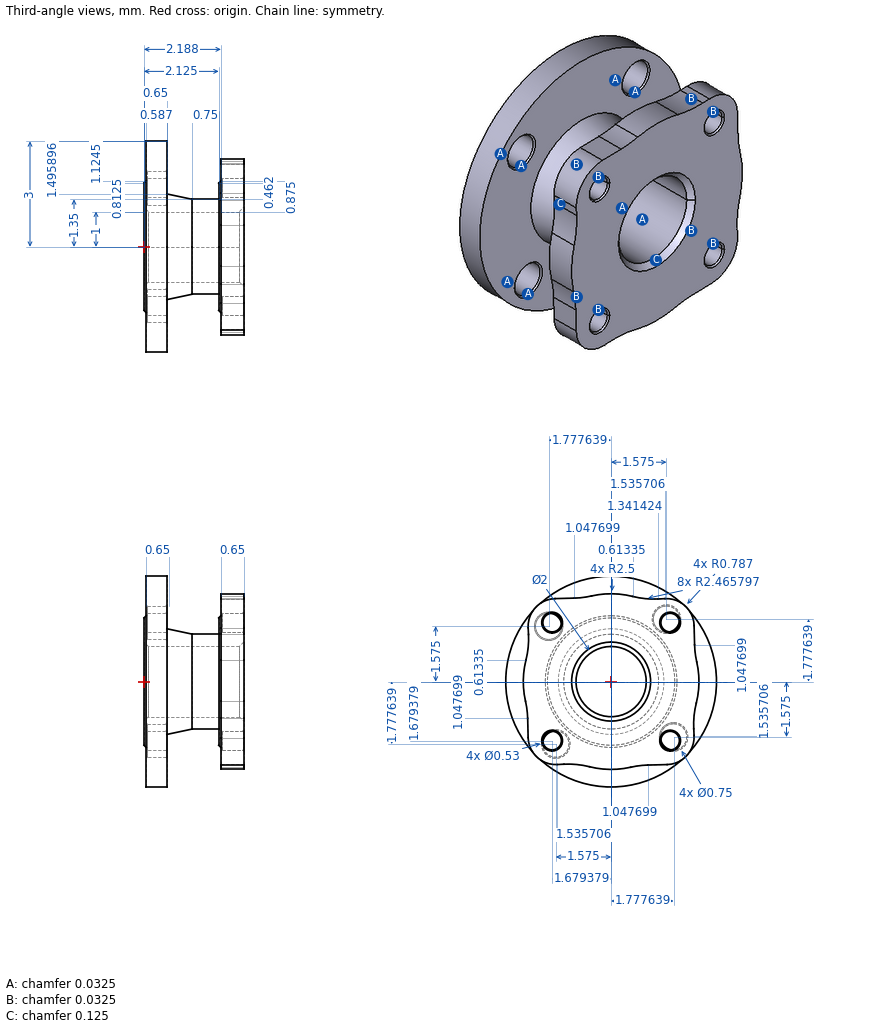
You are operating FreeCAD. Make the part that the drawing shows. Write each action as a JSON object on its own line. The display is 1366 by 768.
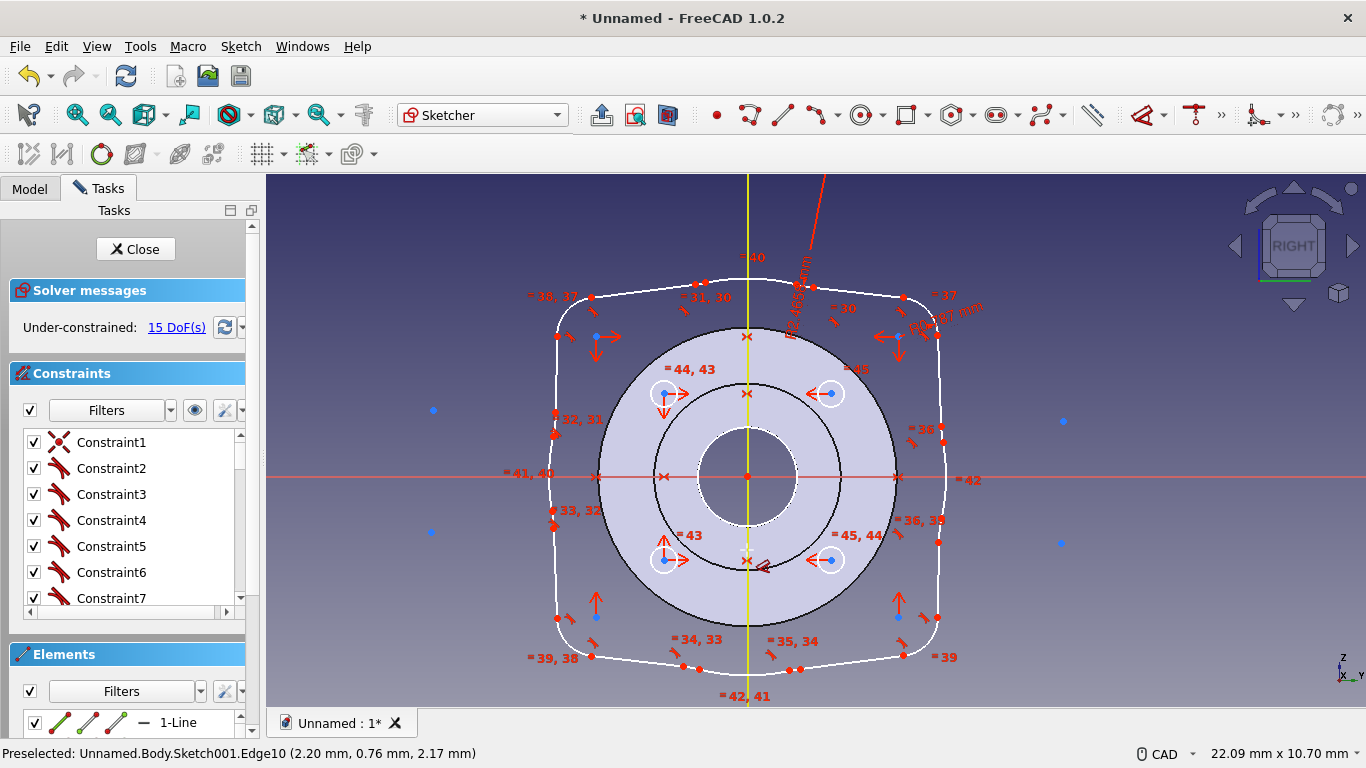
{"action": "left_click", "coordinate": [770, 280]}
{"action": "left_click", "coordinate": [774, 248]}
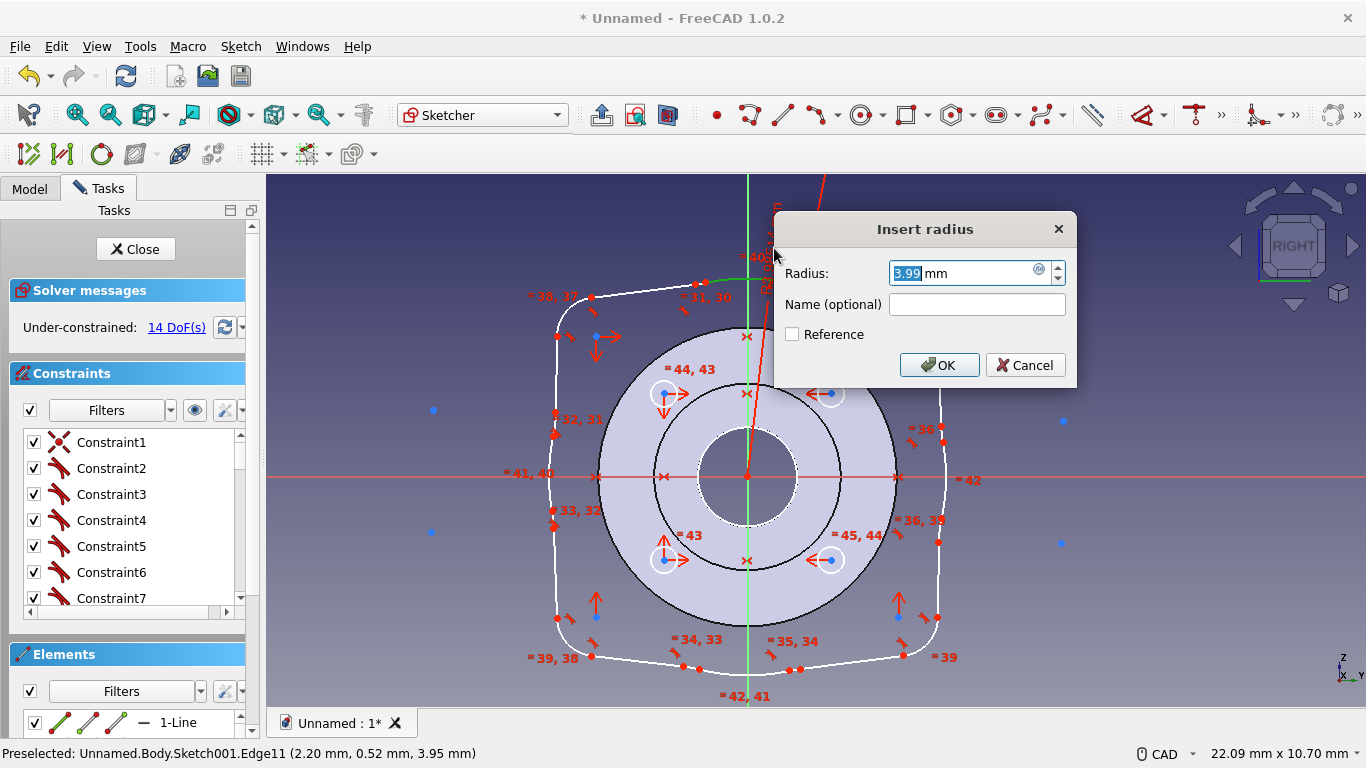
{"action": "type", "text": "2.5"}
{"action": "key", "text": "Return"}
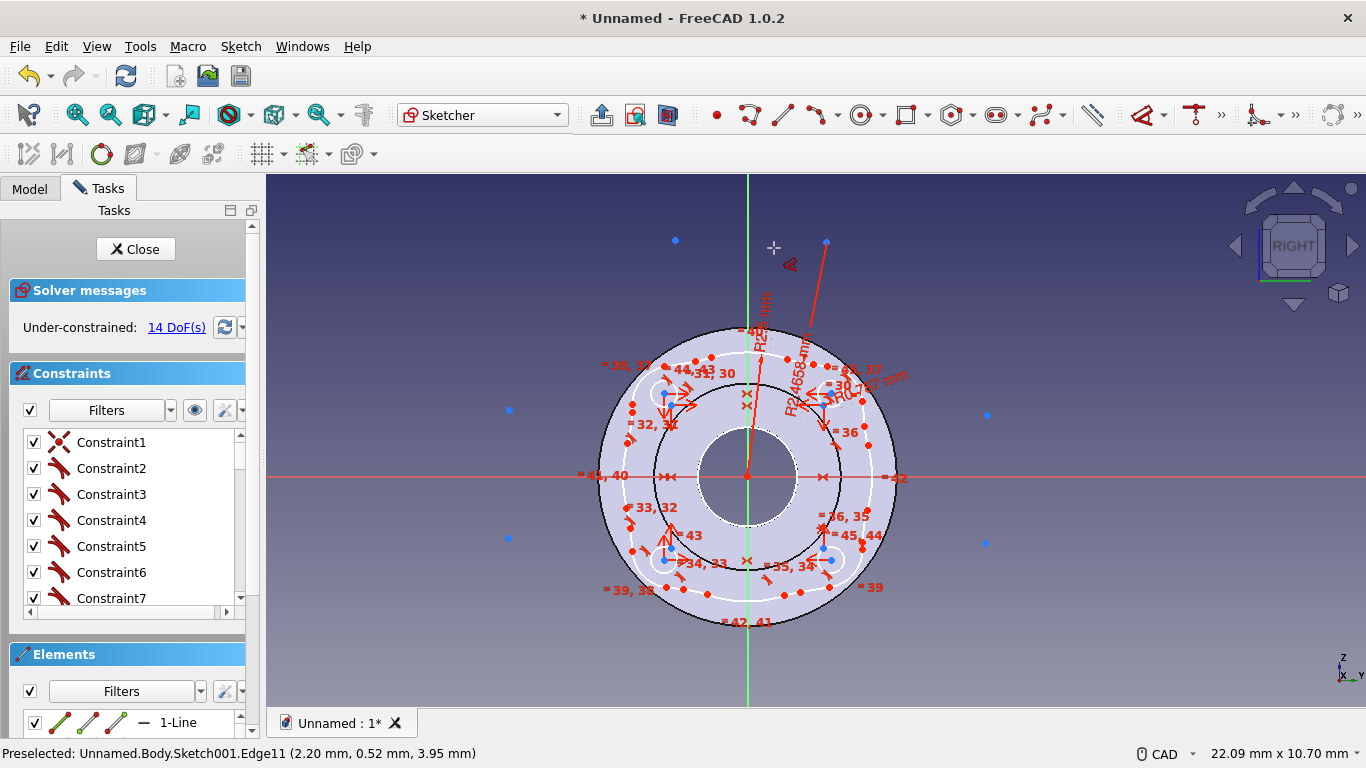
{"action": "scroll", "coordinate": [673, 551], "scroll_direction": "up", "scroll_amount": 3}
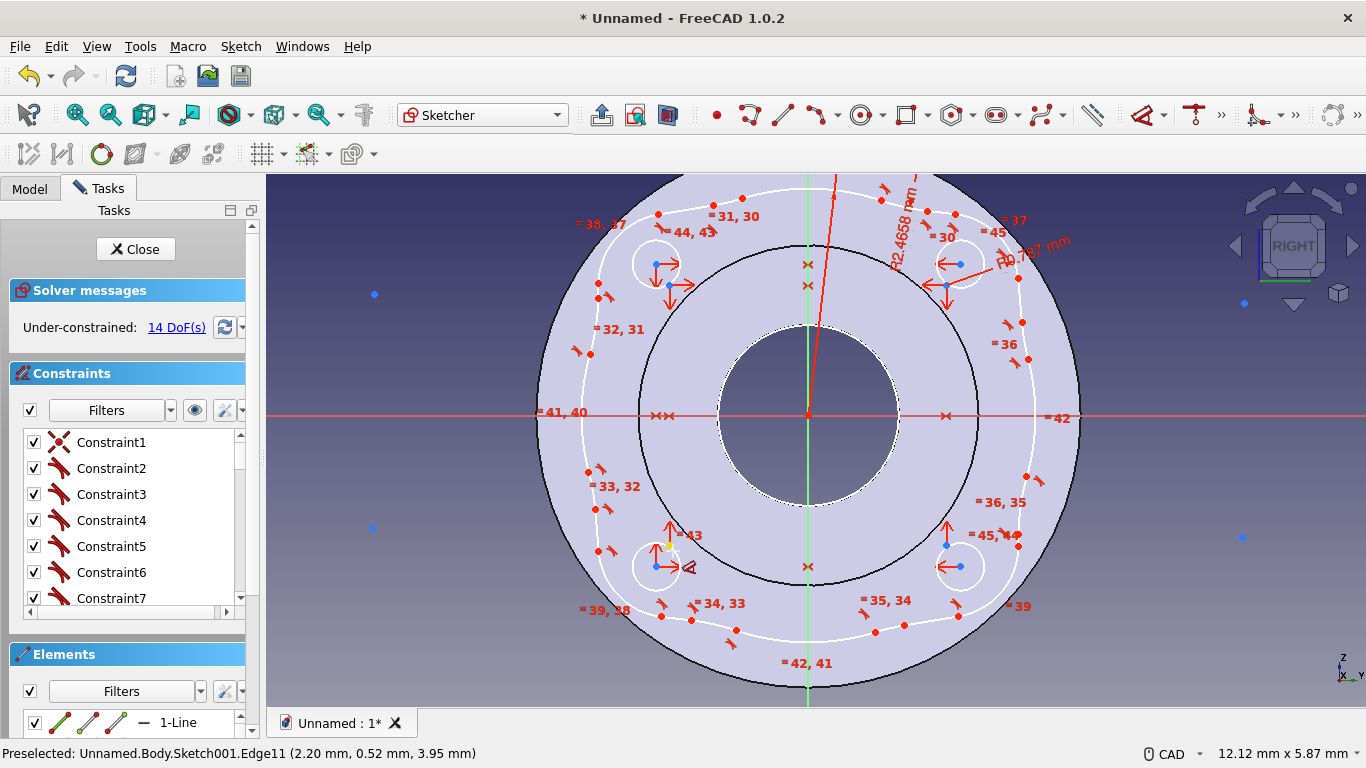
{"action": "left_click", "coordinate": [673, 550]}
{"action": "left_click", "coordinate": [695, 527]}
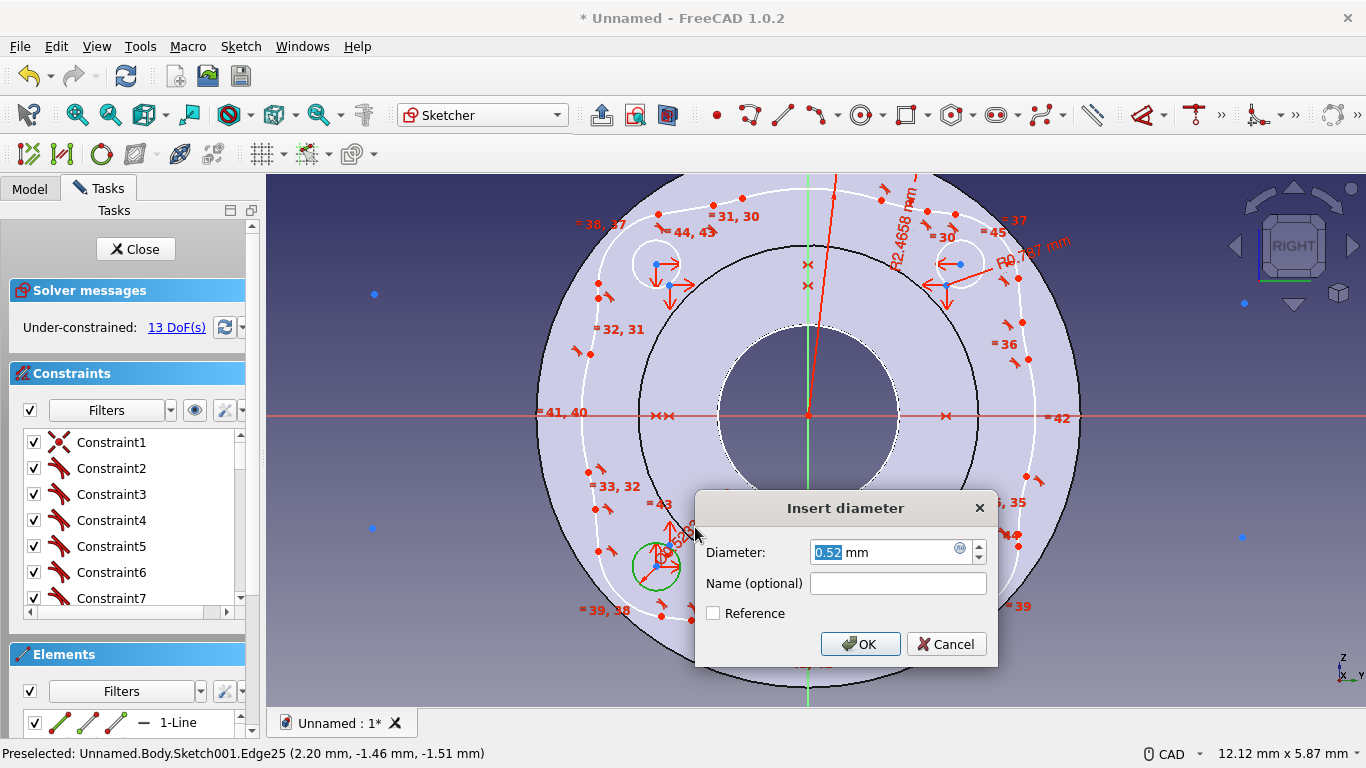
{"action": "type", "text": "0.53"}
{"action": "key", "text": "Return"}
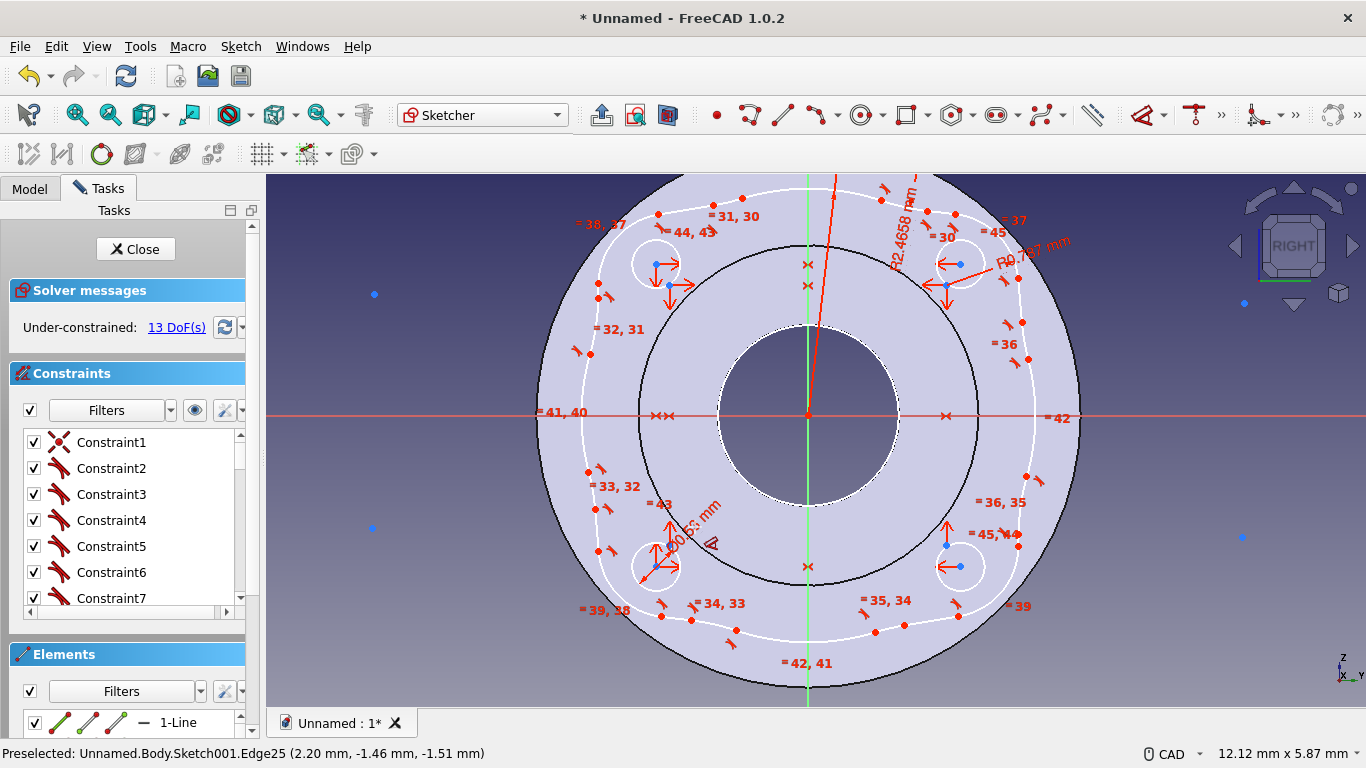
{"action": "left_click", "coordinate": [872, 351]}
{"action": "left_click", "coordinate": [894, 328]}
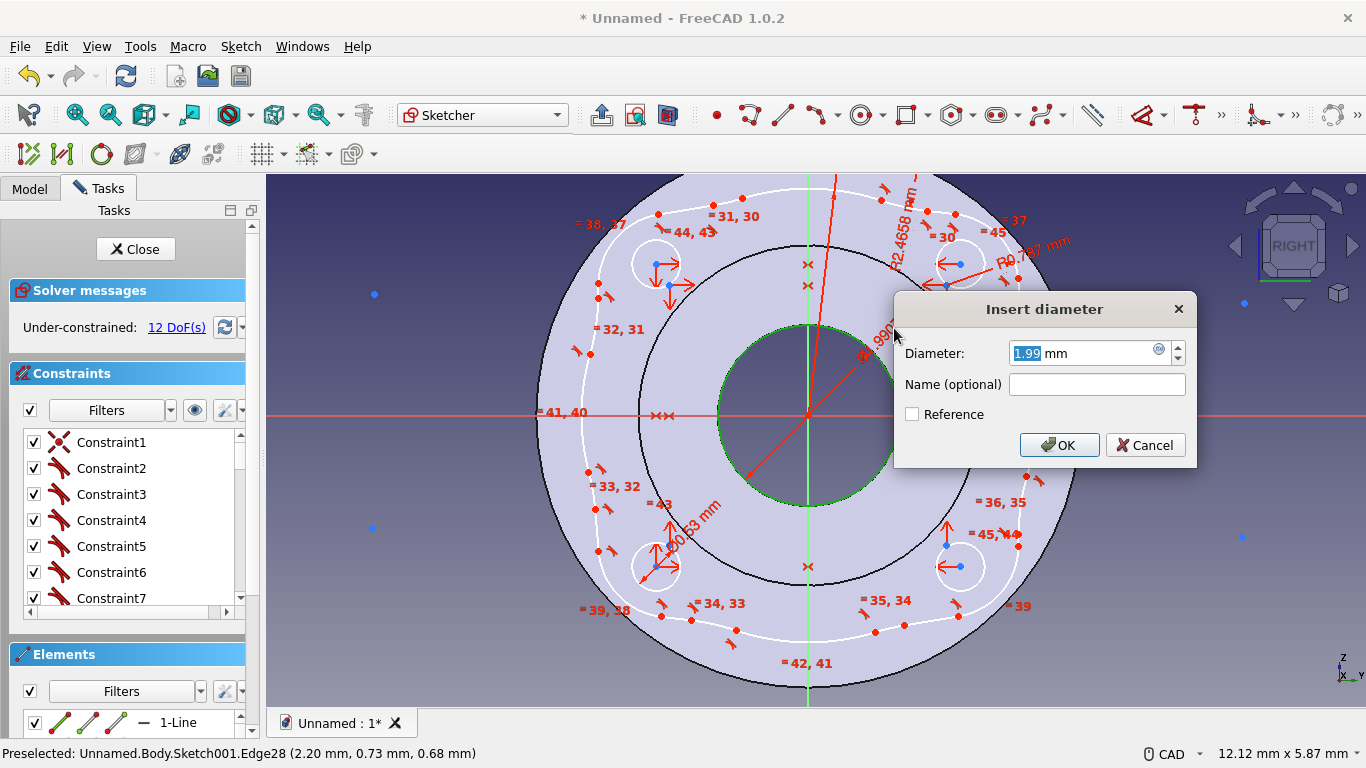
{"action": "type", "text": "2"}
{"action": "key", "text": "Return"}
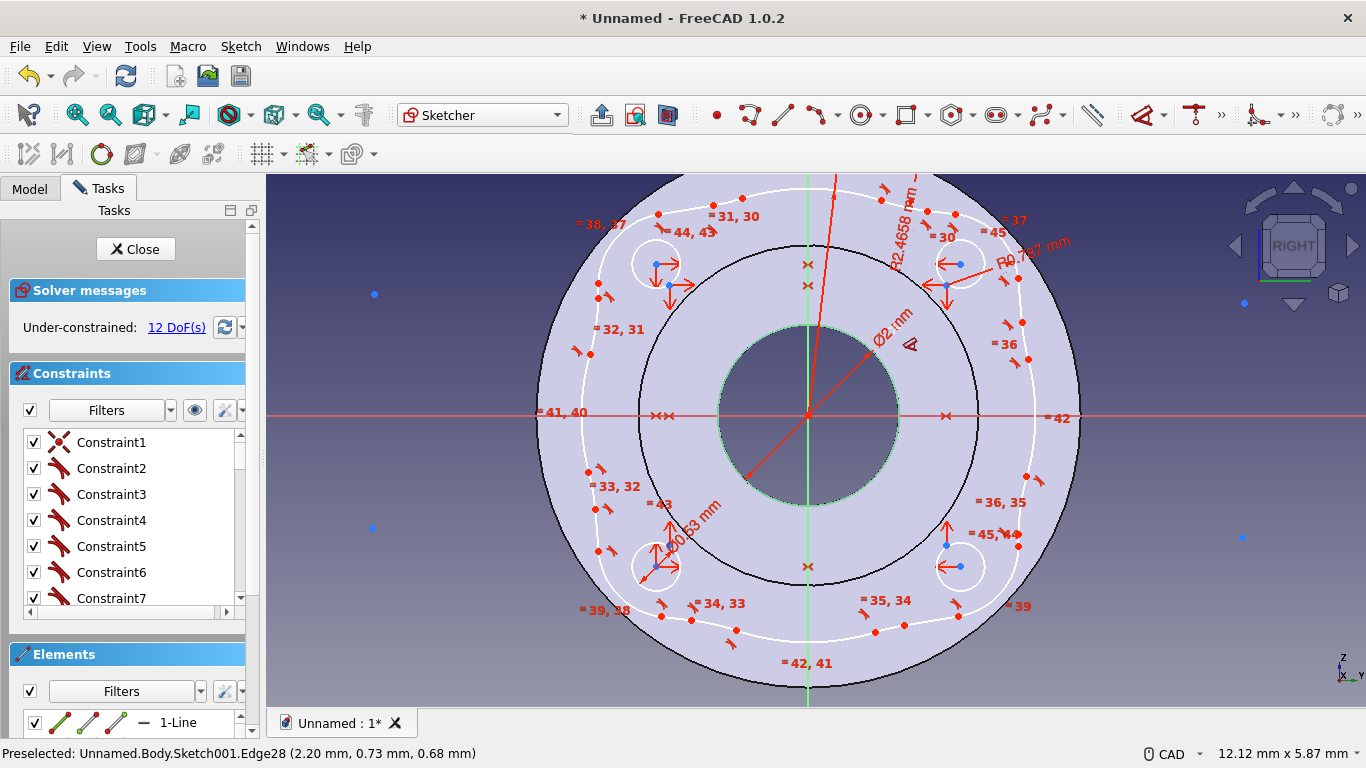
{"action": "scroll", "coordinate": [472, 553], "scroll_direction": "down", "scroll_amount": 1}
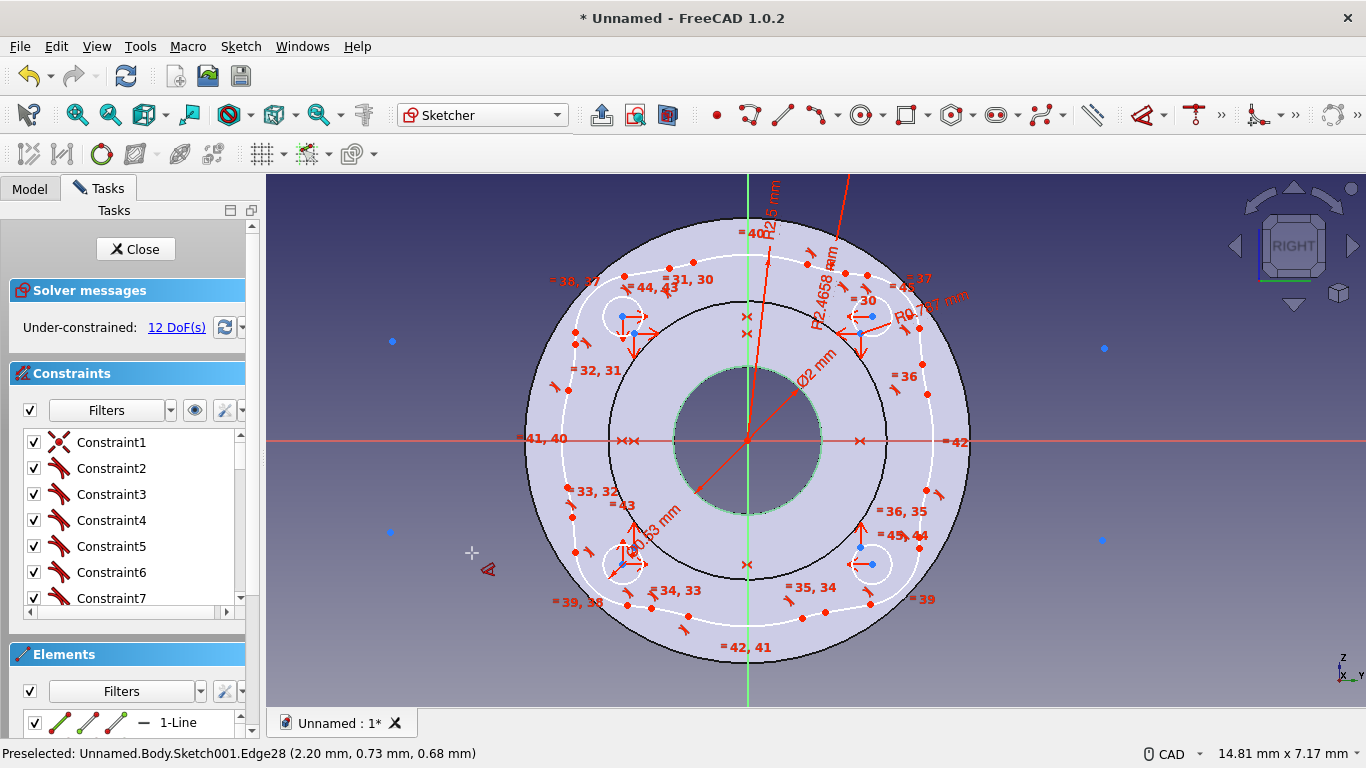
{"action": "left_click", "coordinate": [807, 265]}
{"action": "left_click", "coordinate": [777, 231]}